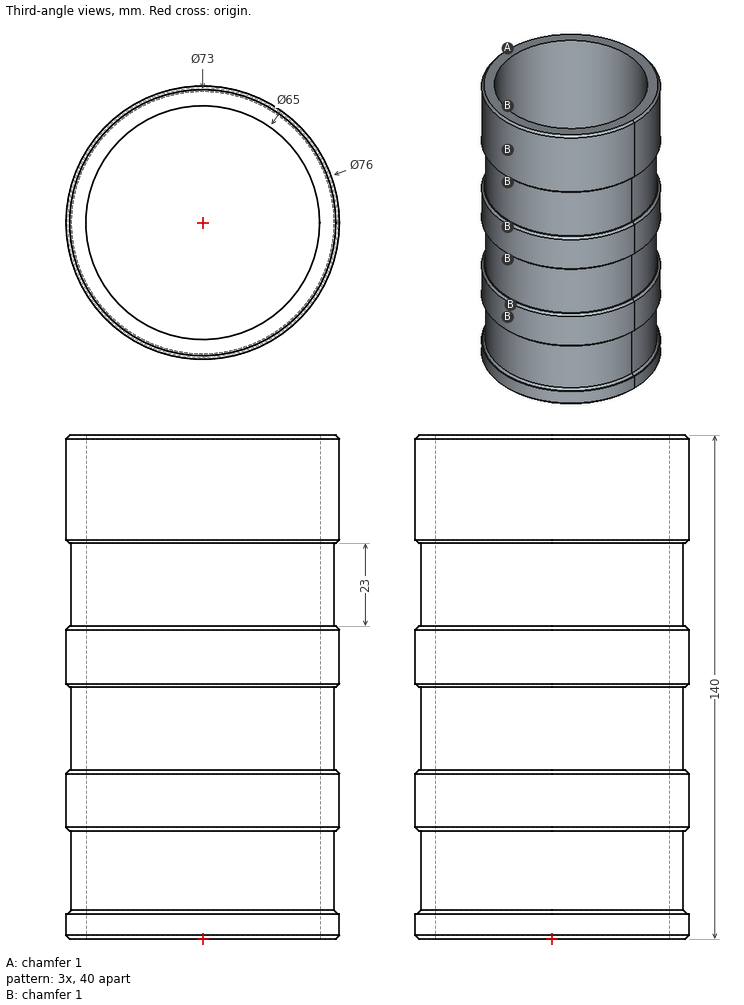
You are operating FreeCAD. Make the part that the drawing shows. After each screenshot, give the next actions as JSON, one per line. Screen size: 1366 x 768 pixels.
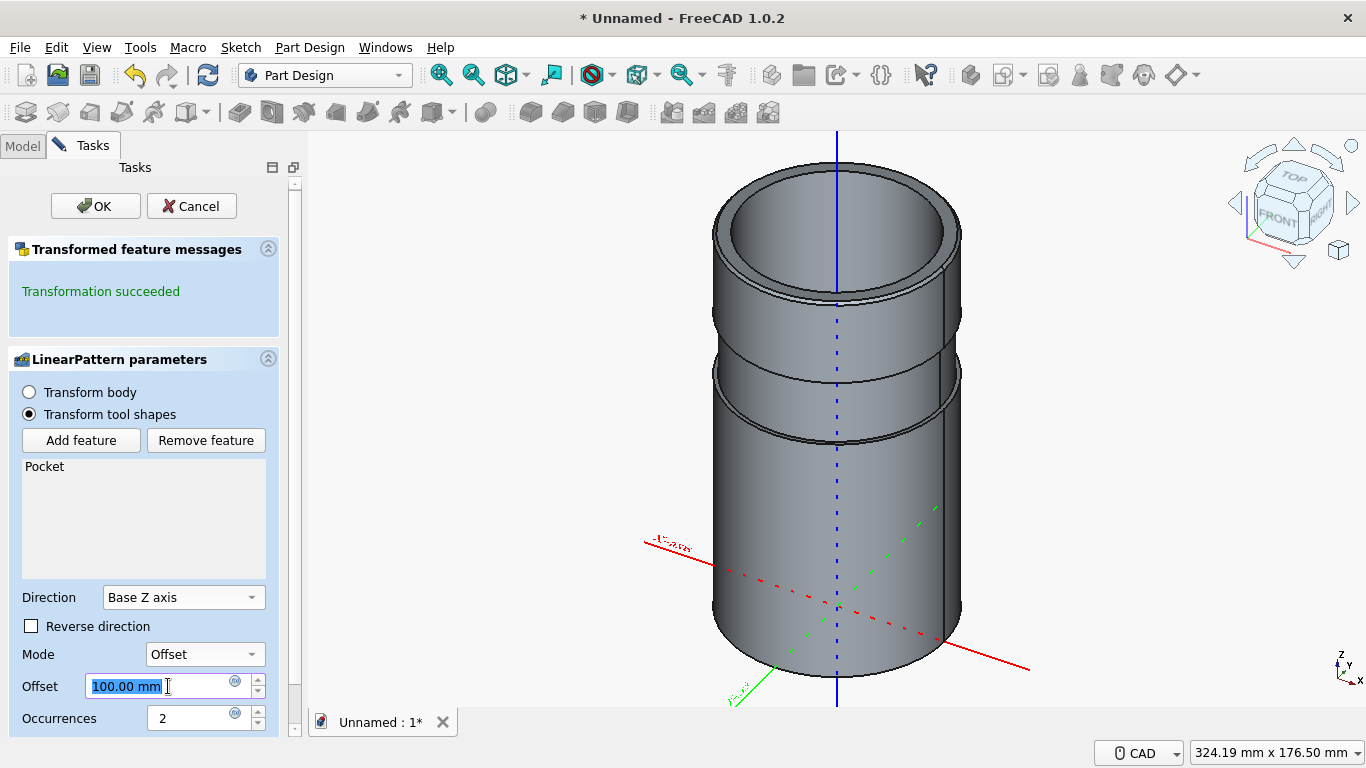
{"action": "type", "text": "40"}
{"action": "key", "text": "Tab"}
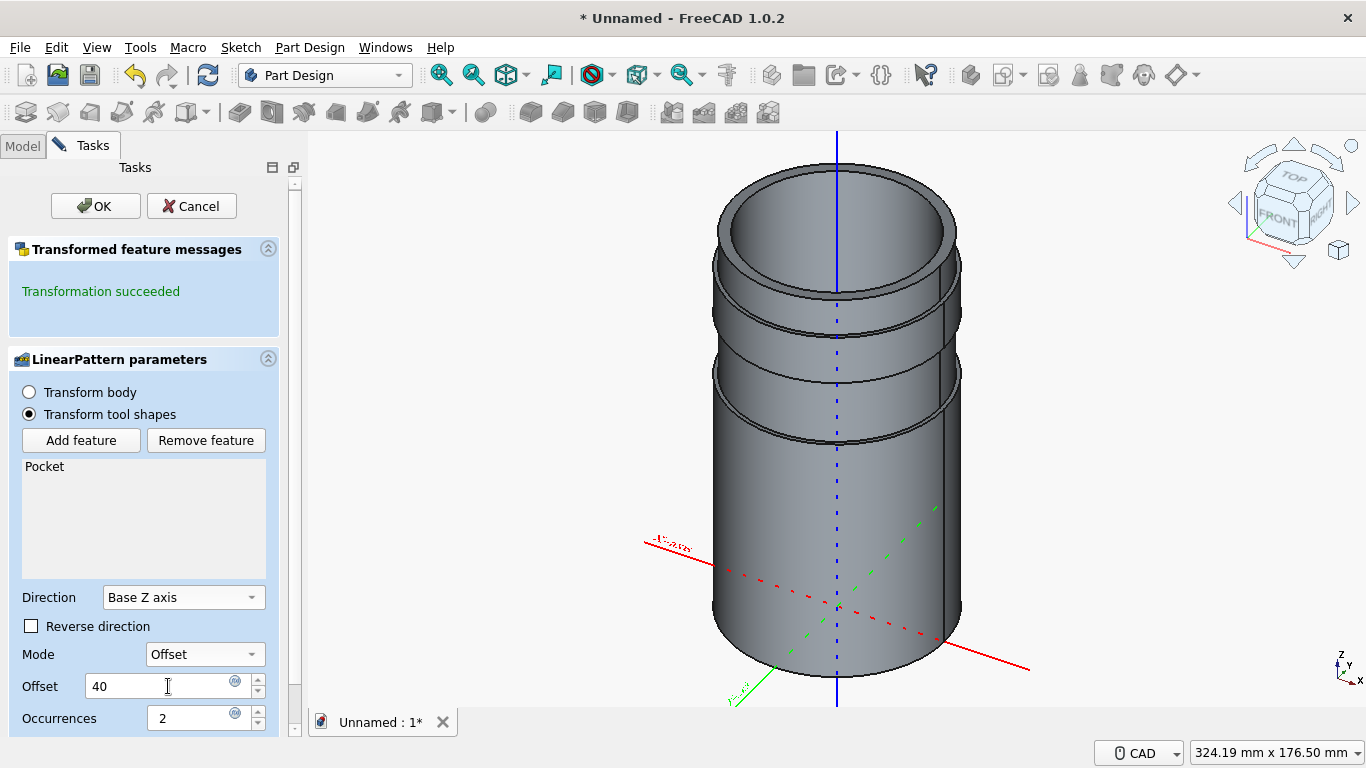
{"action": "triple_click", "coordinate": [198, 718]}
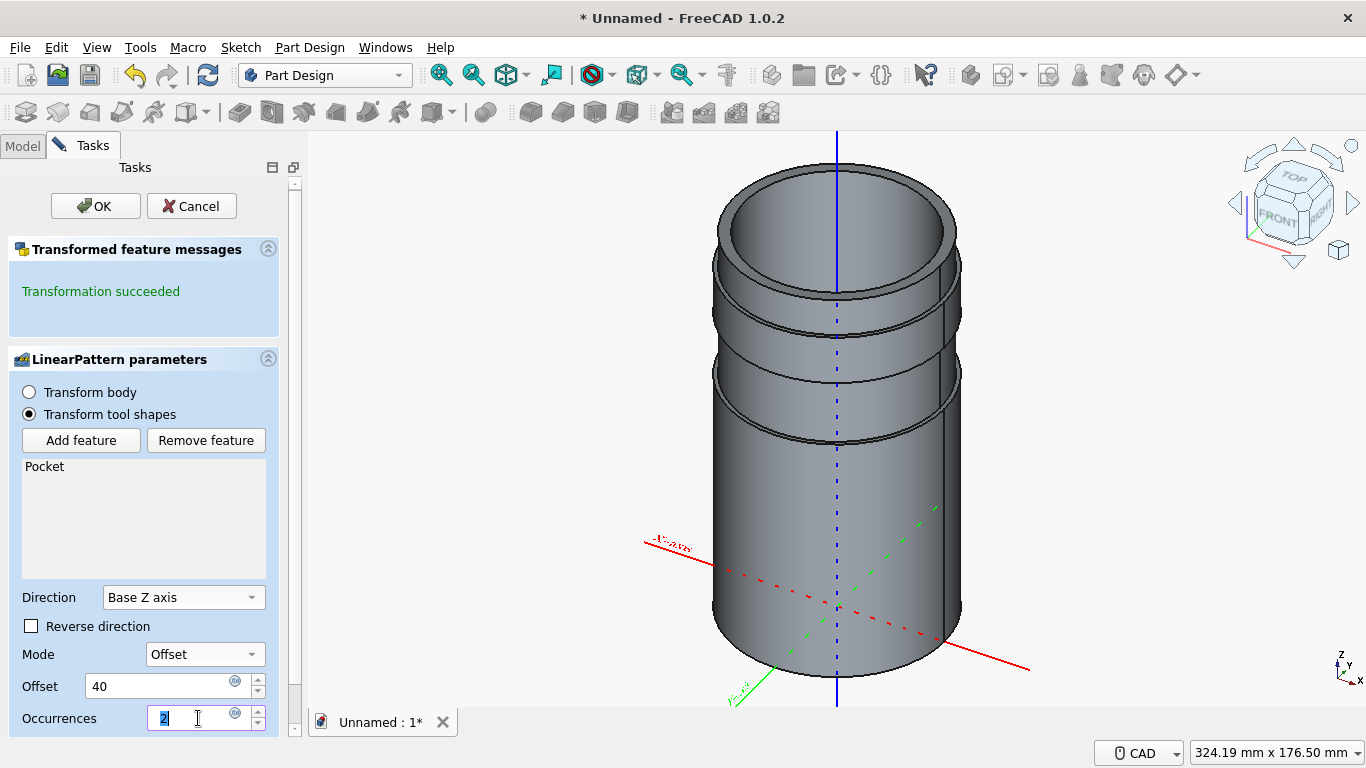
{"action": "type", "text": "3"}
{"action": "key", "text": "Tab"}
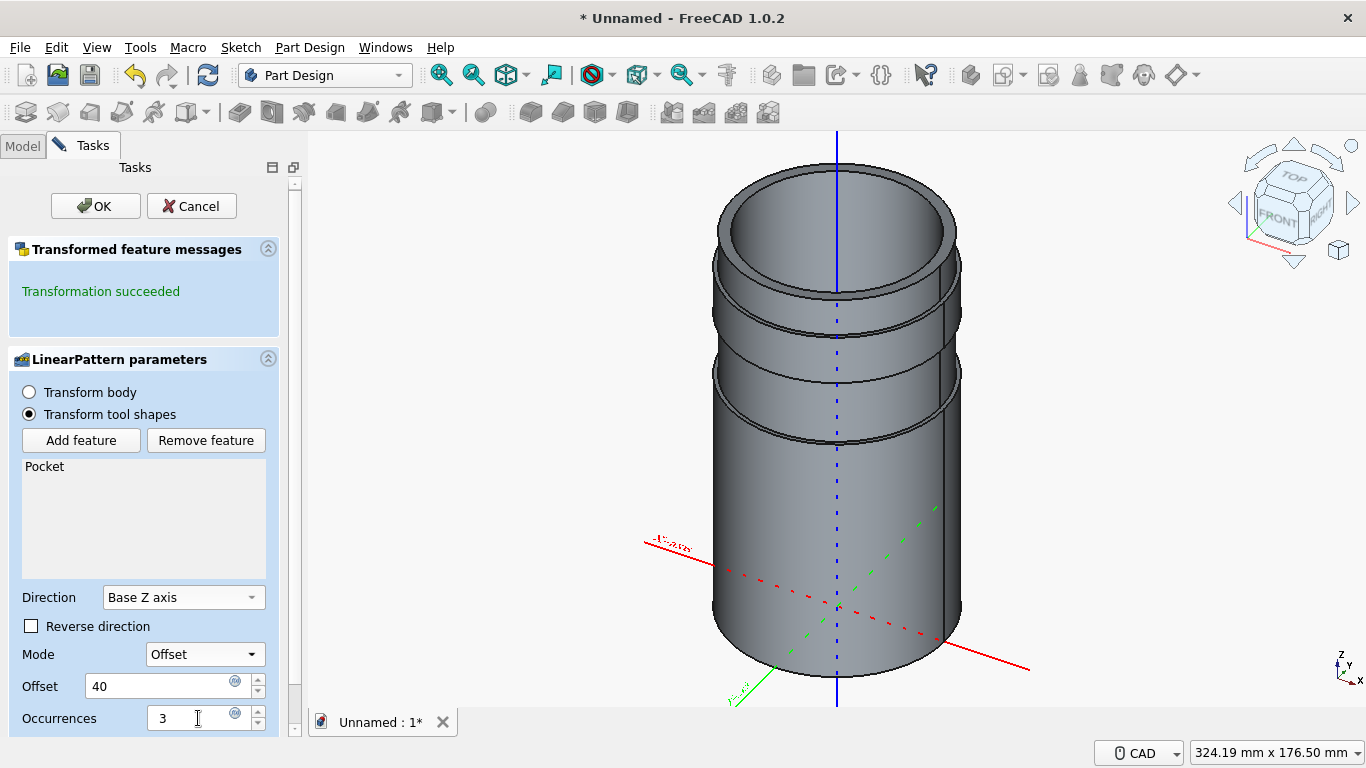
{"action": "left_click", "coordinate": [30, 626]}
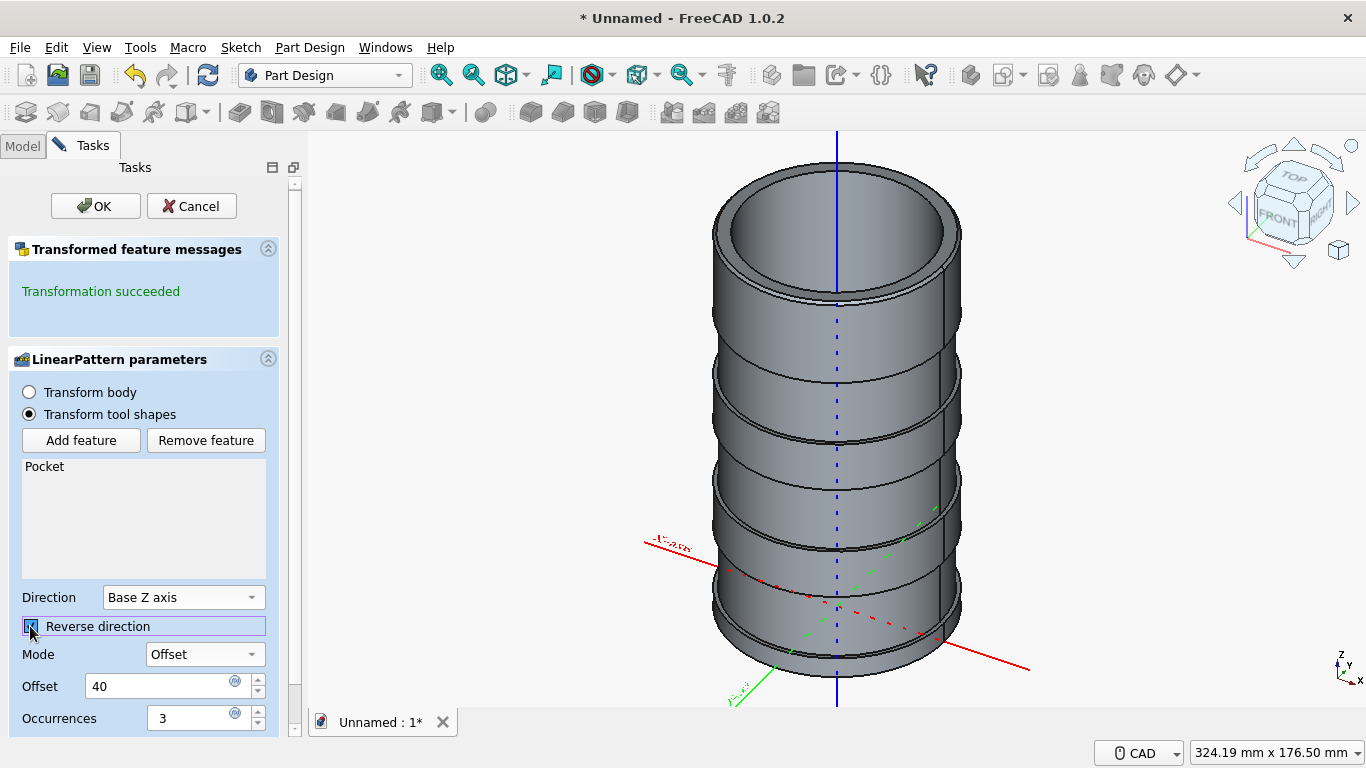
{"action": "left_click", "coordinate": [96, 206]}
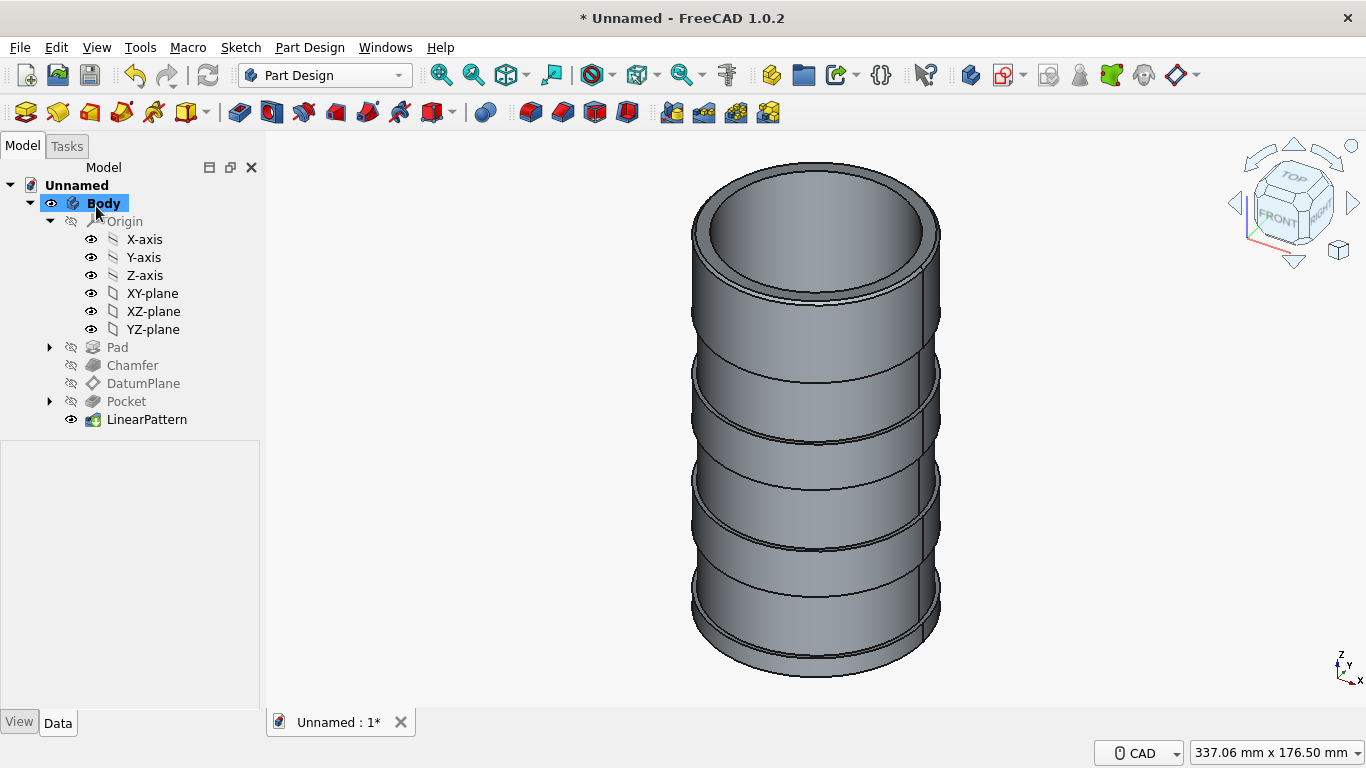
{"action": "left_click", "coordinate": [693, 380]}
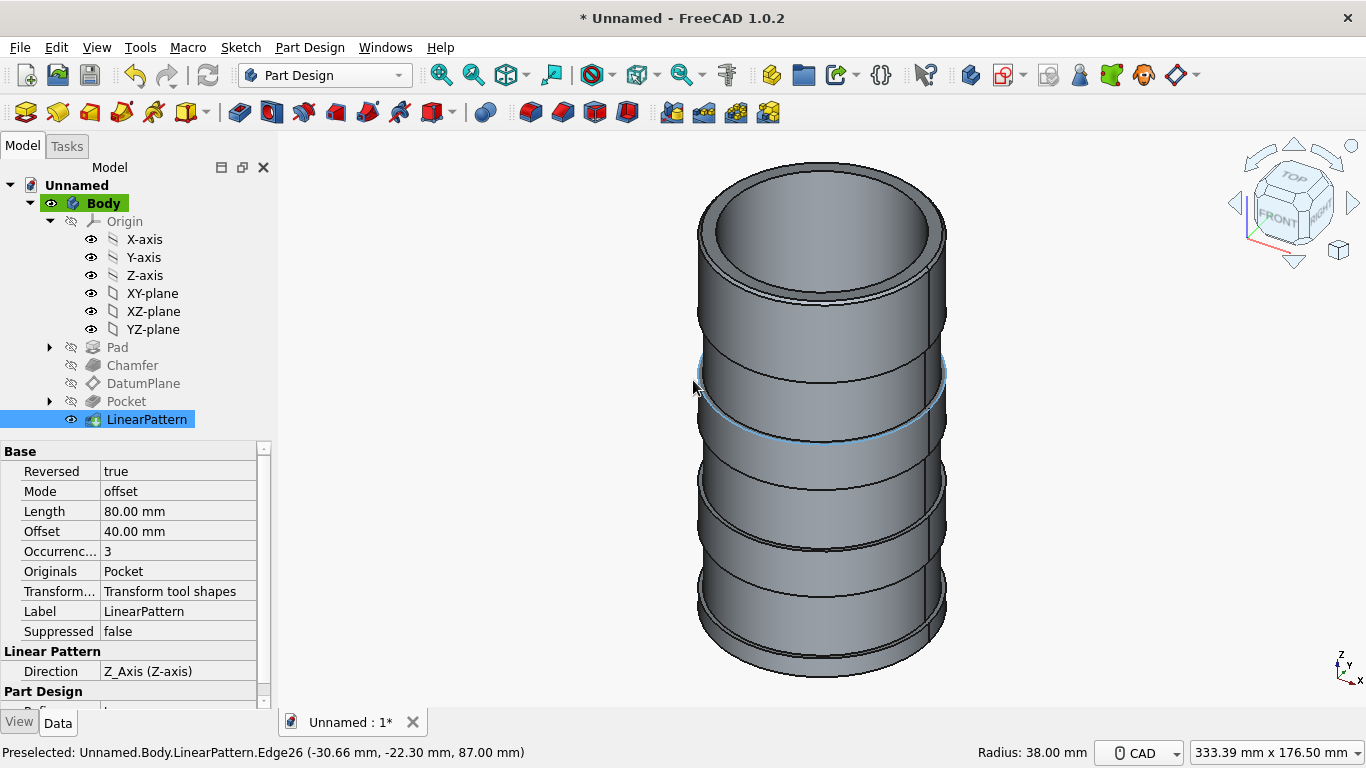
{"action": "left_click", "coordinate": [730, 359], "text": "ctrl"}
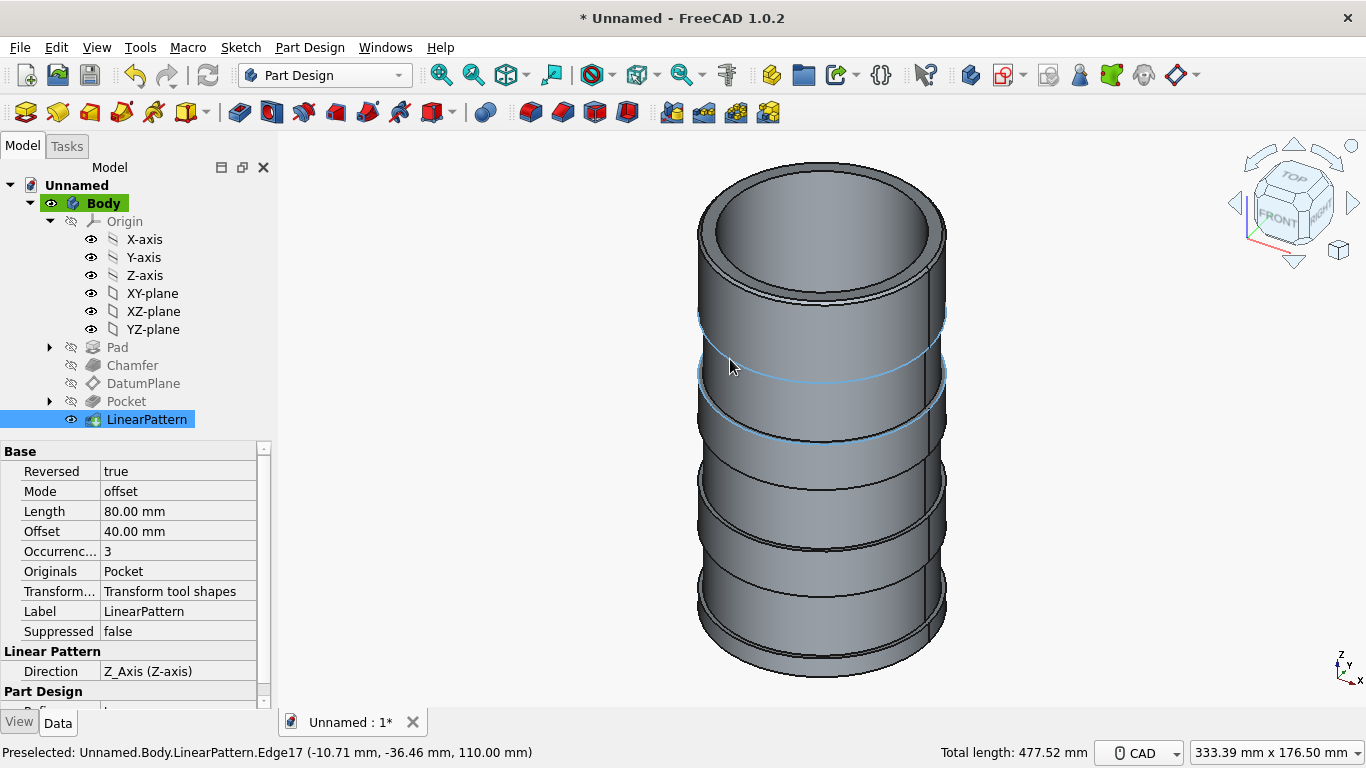
{"action": "left_click", "coordinate": [730, 653], "text": "ctrl"}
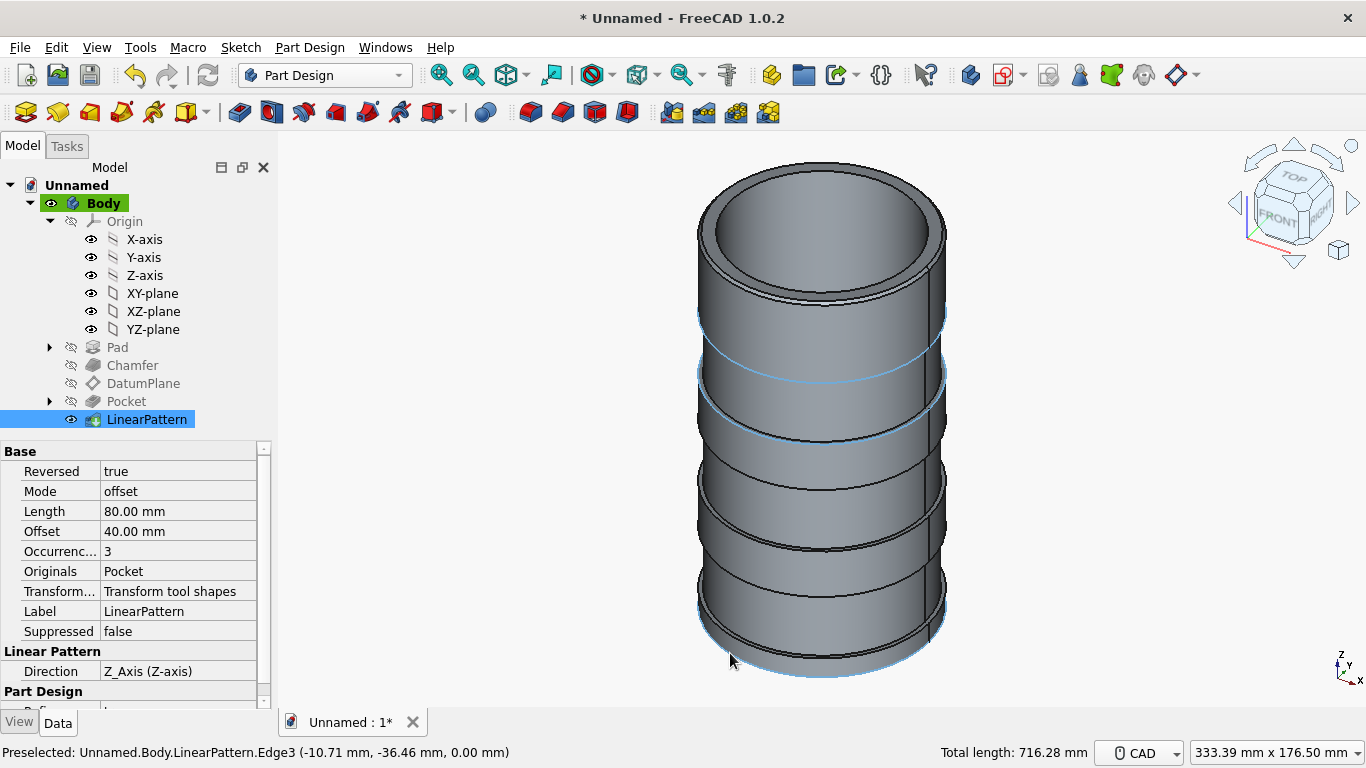
{"action": "left_click", "coordinate": [699, 487], "text": "ctrl"}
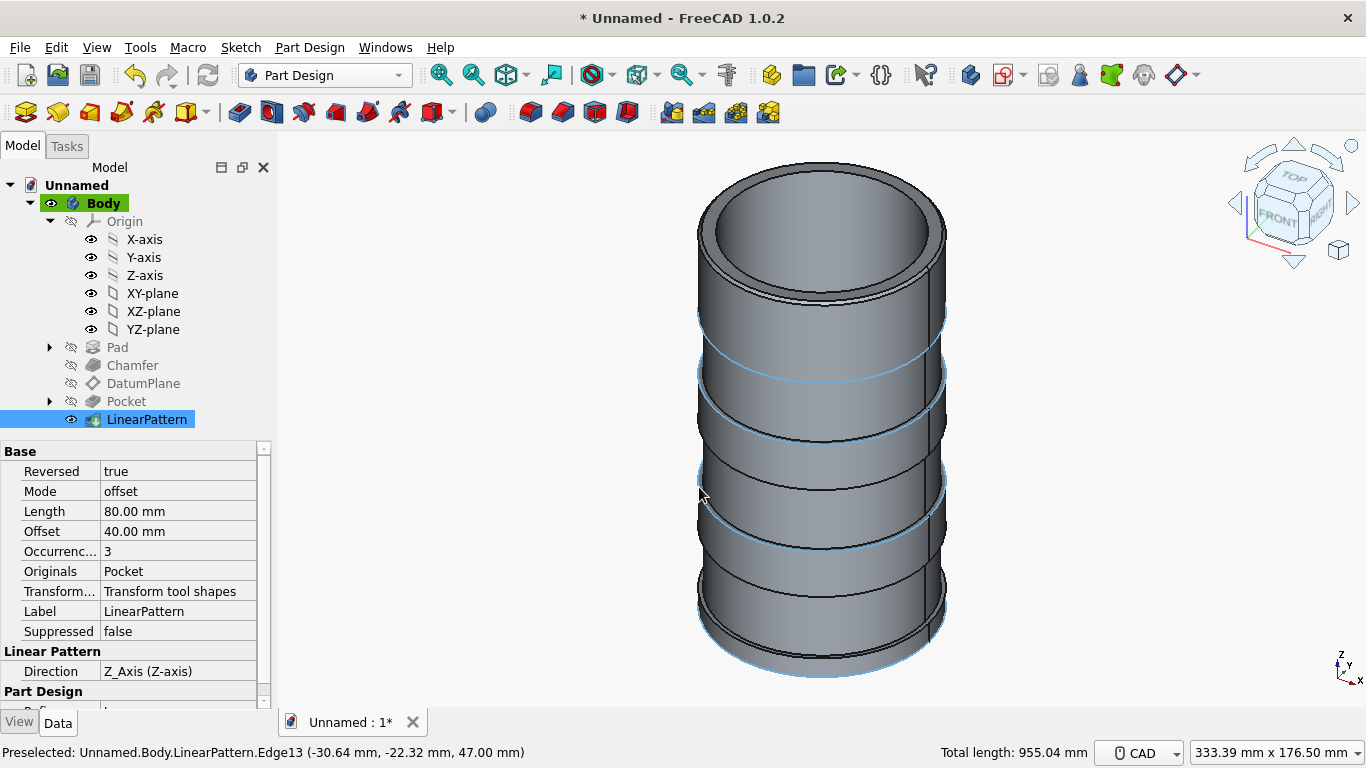
{"action": "left_click", "coordinate": [730, 466], "text": "ctrl"}